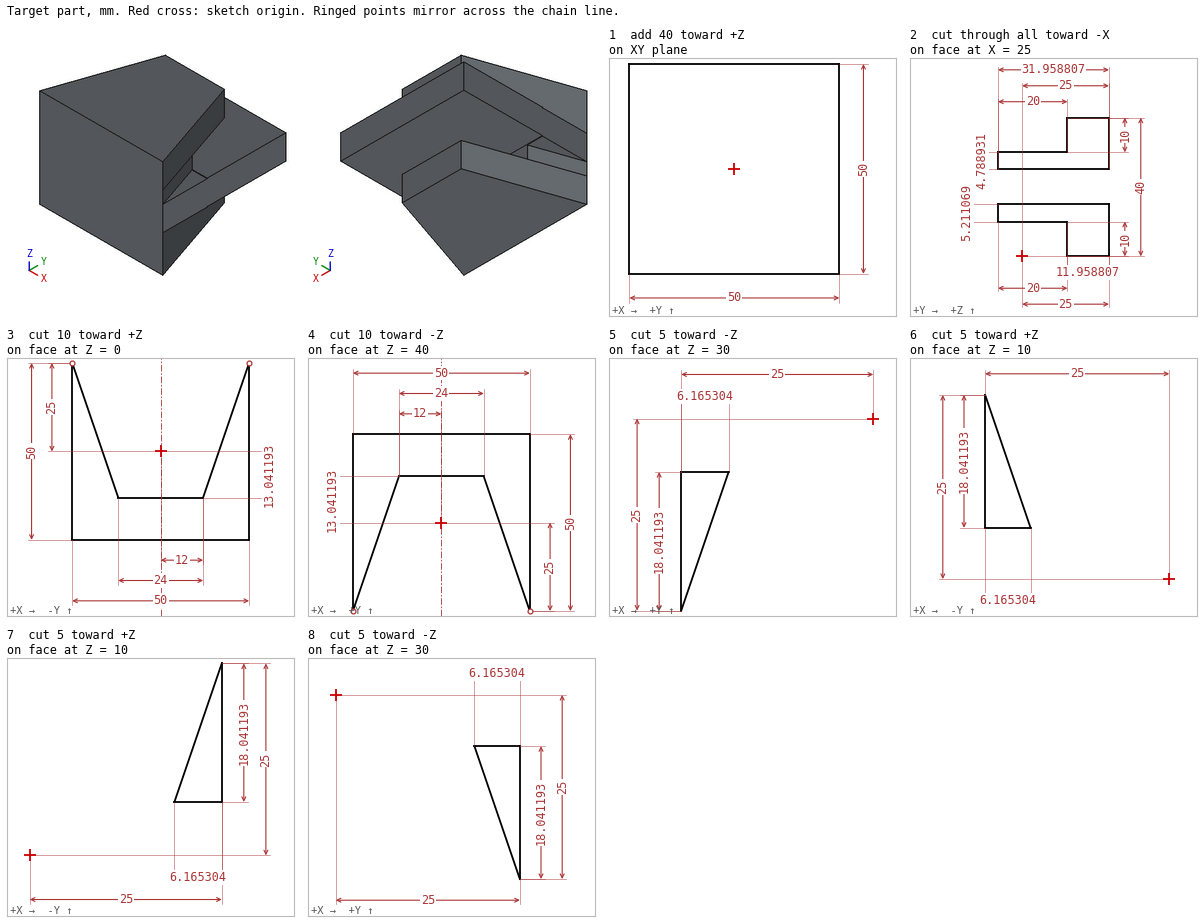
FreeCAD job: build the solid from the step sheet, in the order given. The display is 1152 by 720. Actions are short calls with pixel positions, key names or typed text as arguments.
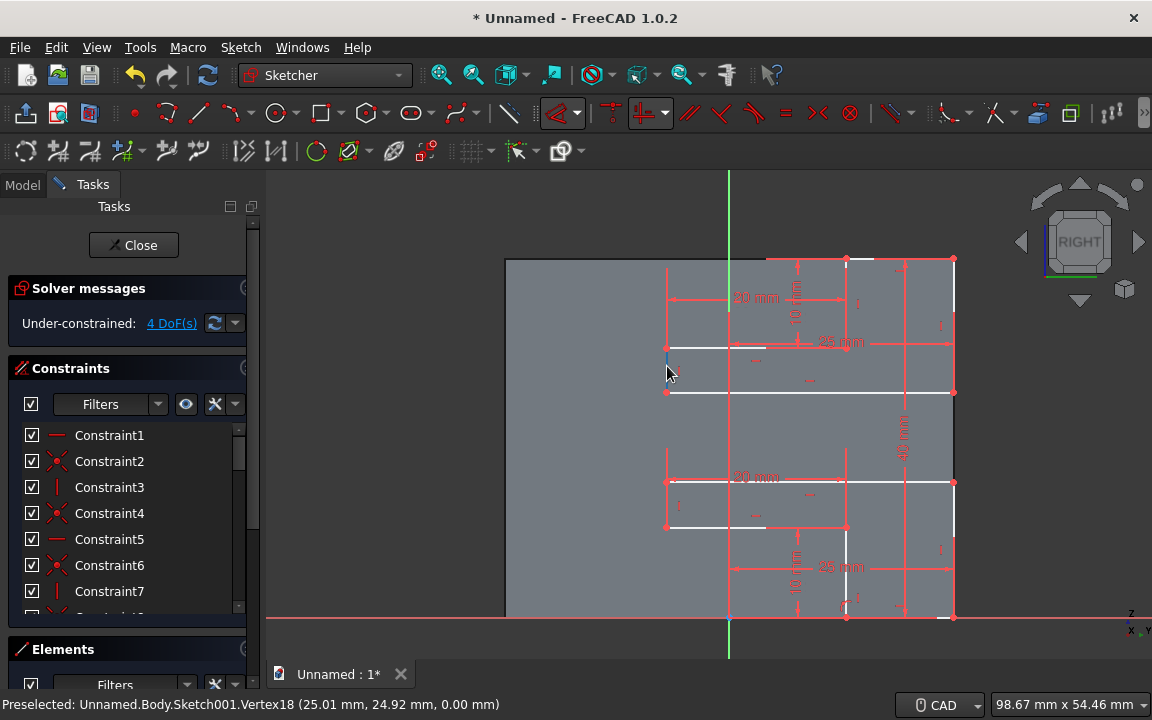
click(667, 366)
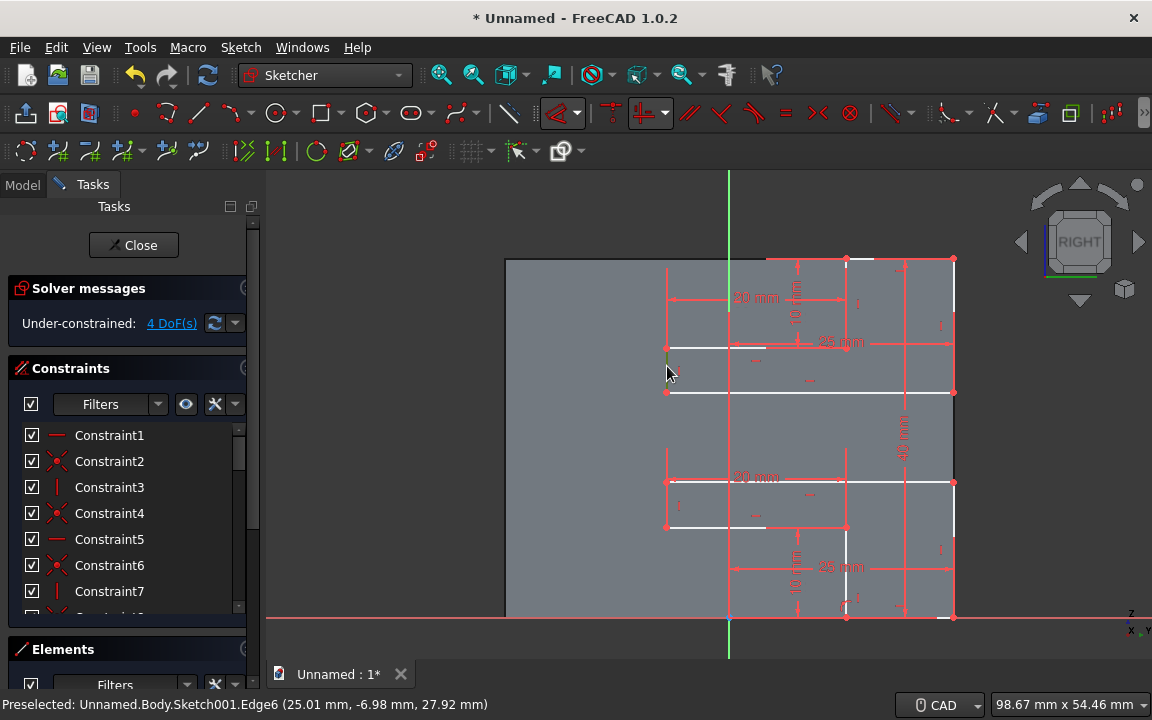
key(i)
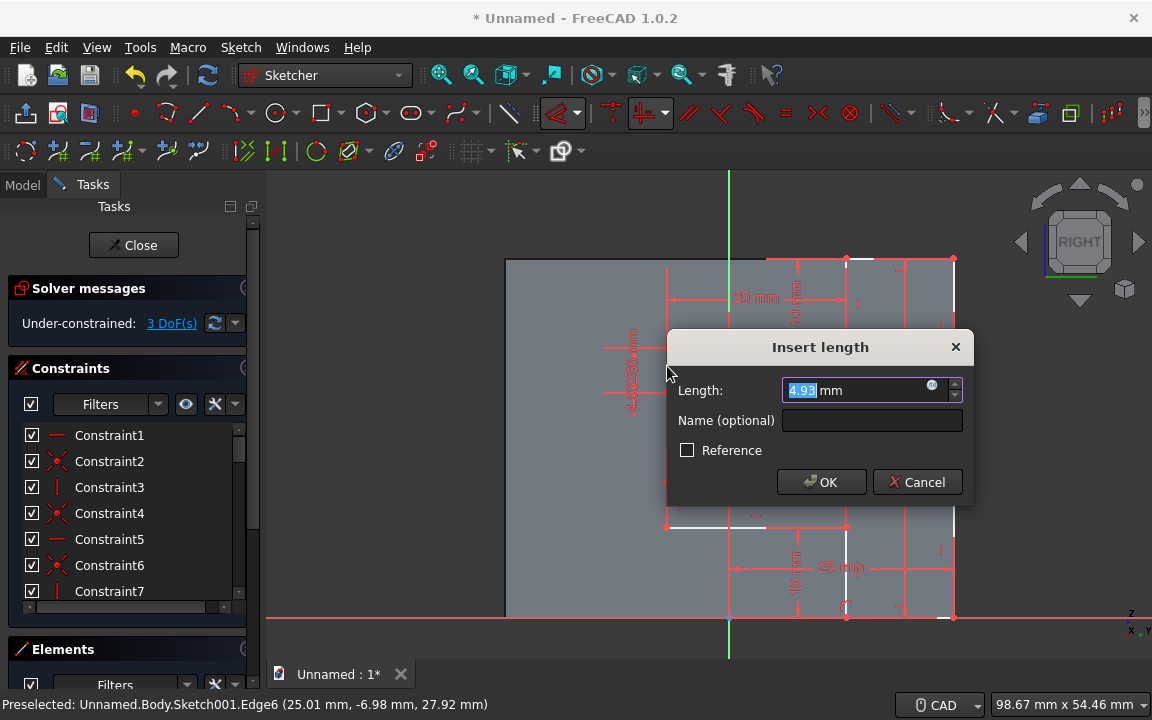
text(4.788931)
key(Return)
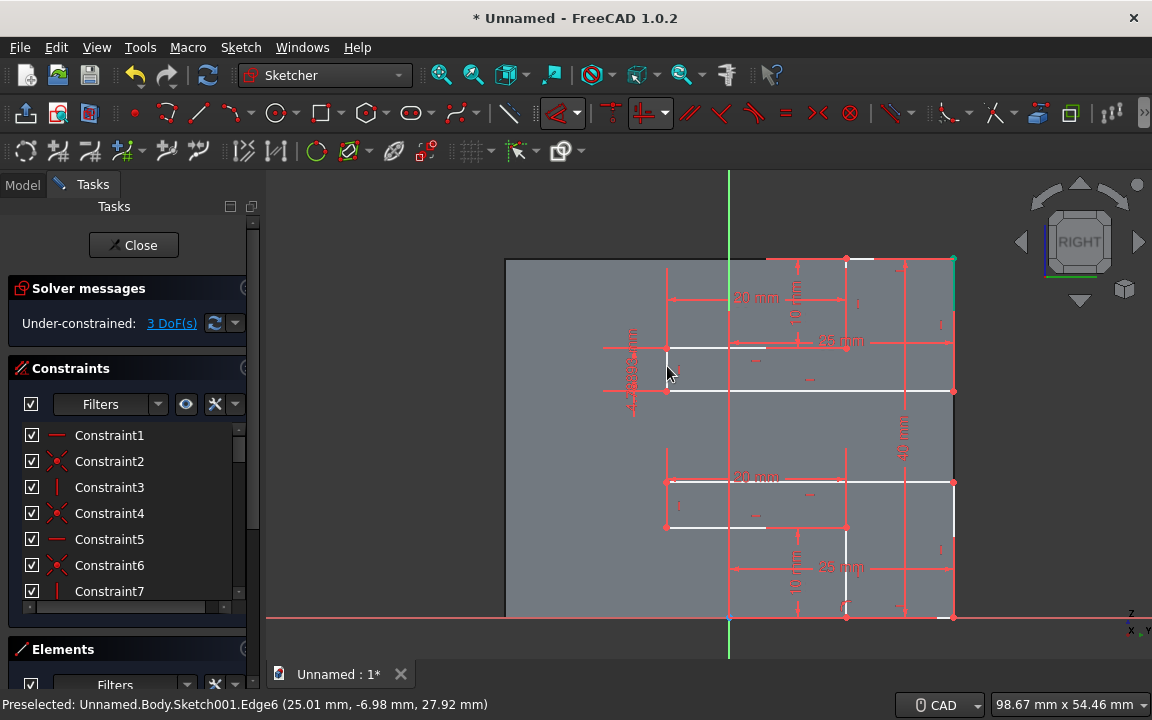
click(667, 496)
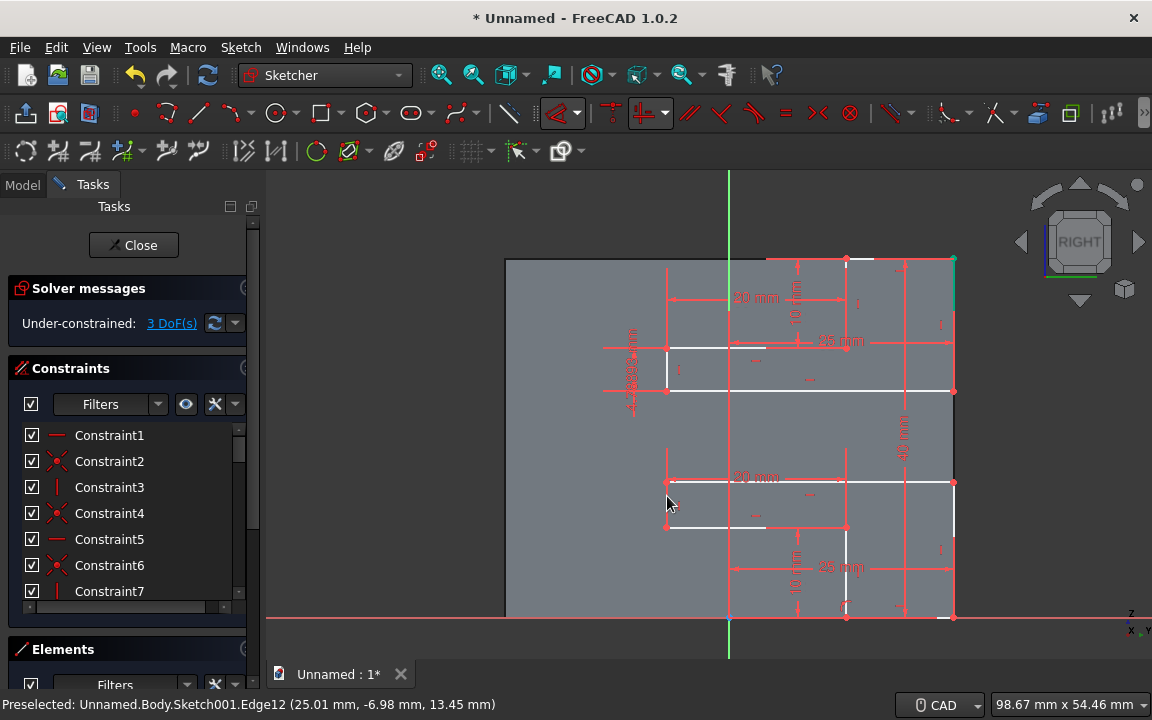
key(i)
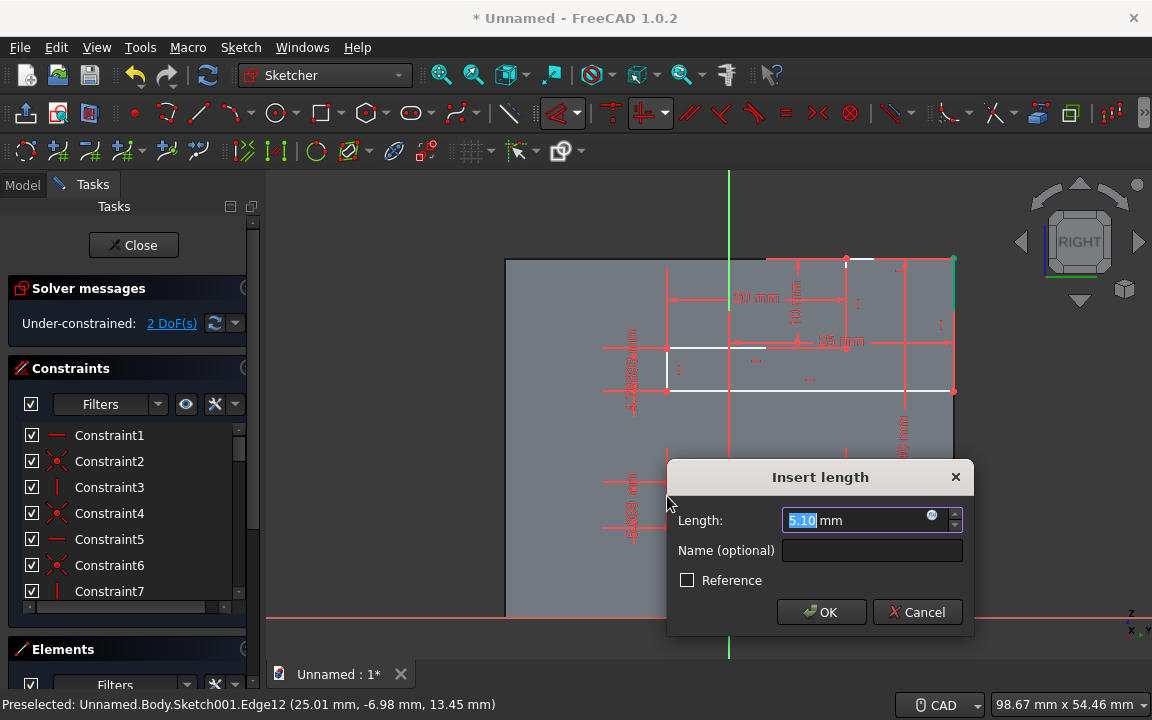
text(5.211069)
key(Return)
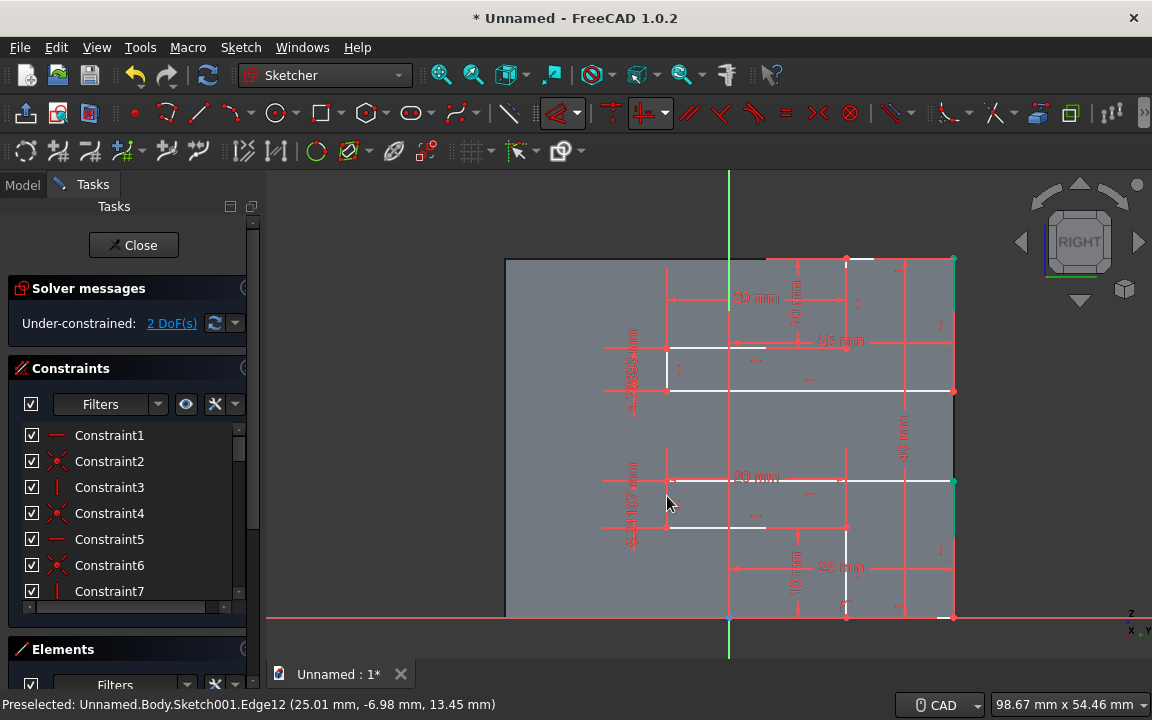
click(753, 391)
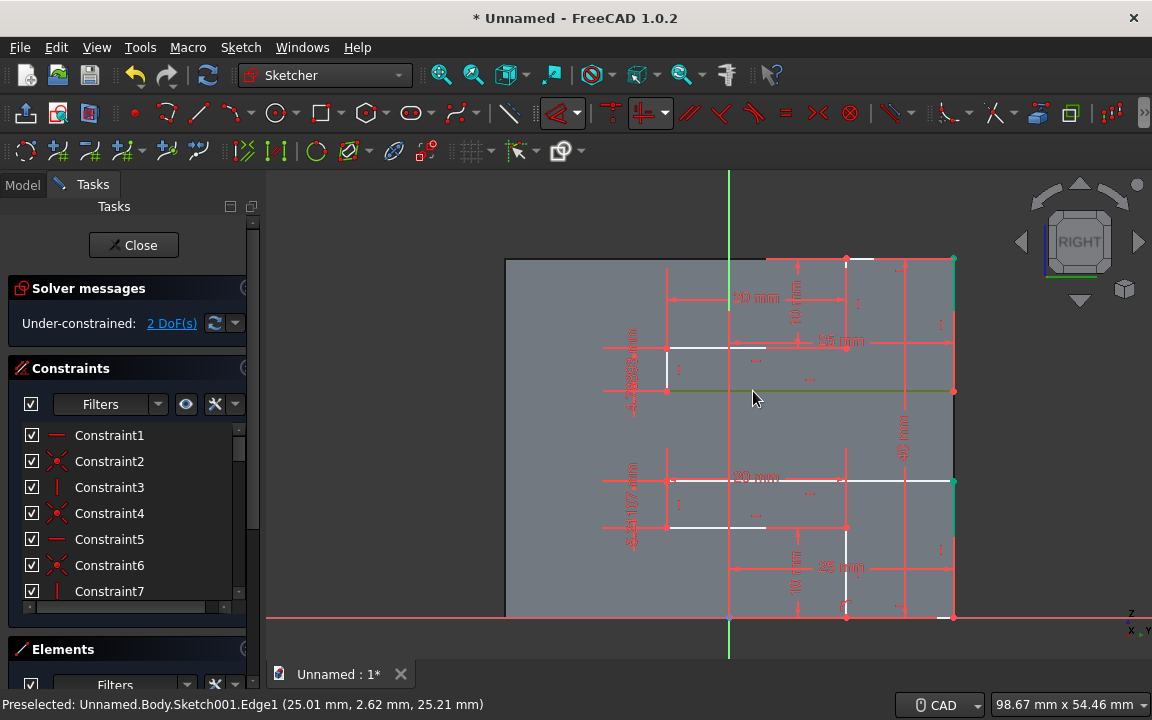
key(l)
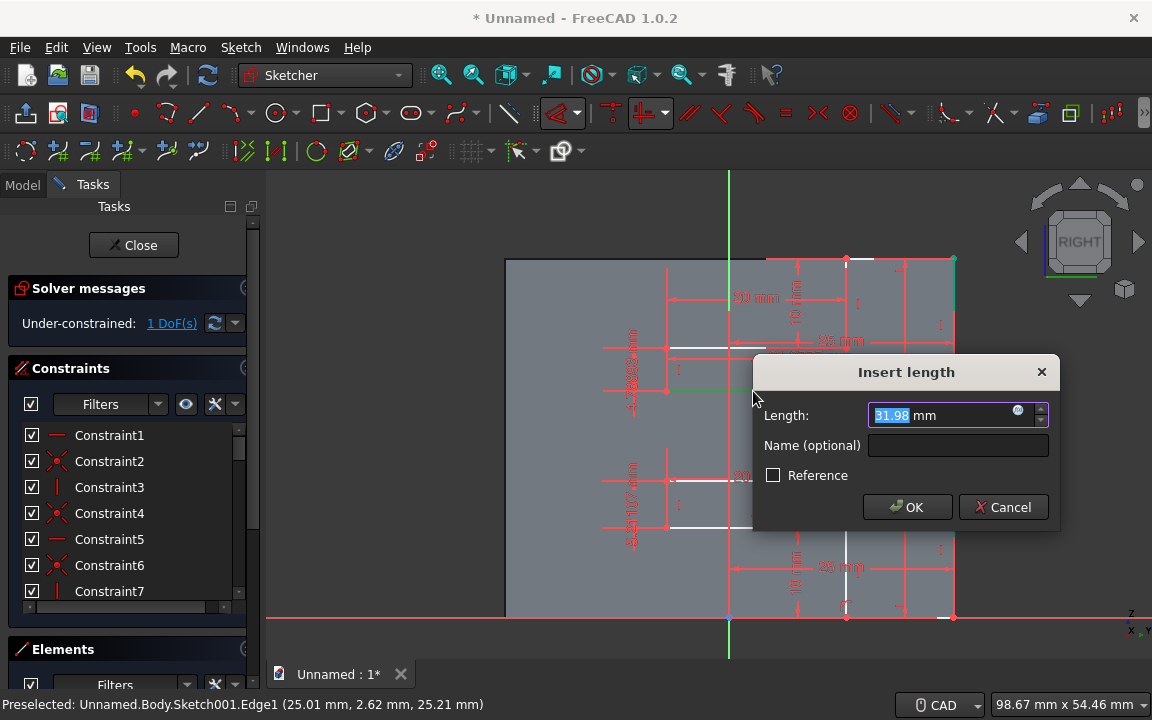
text(31.958807)
key(Return)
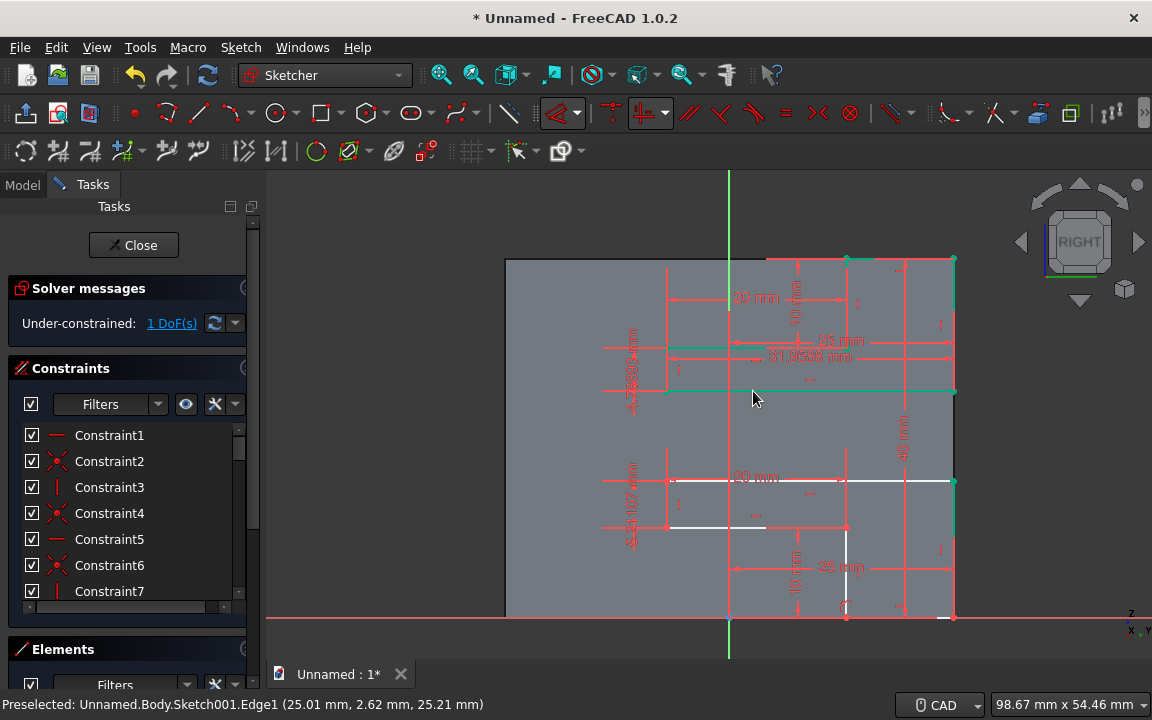
click(879, 618)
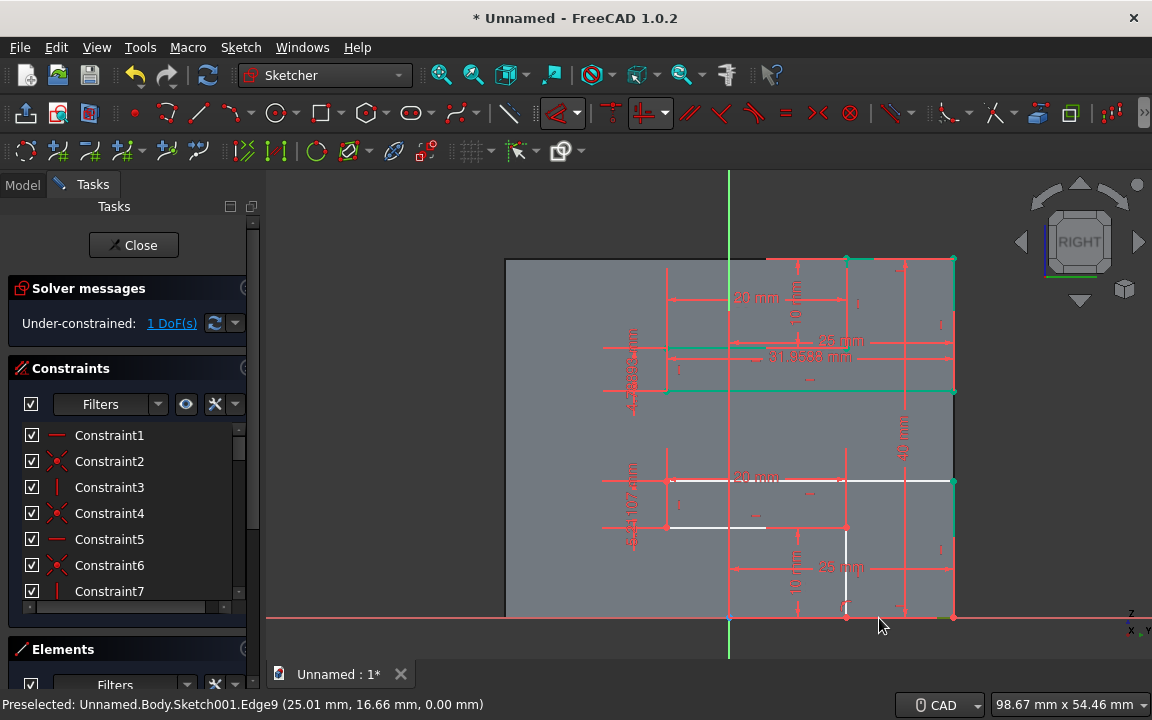
key(l)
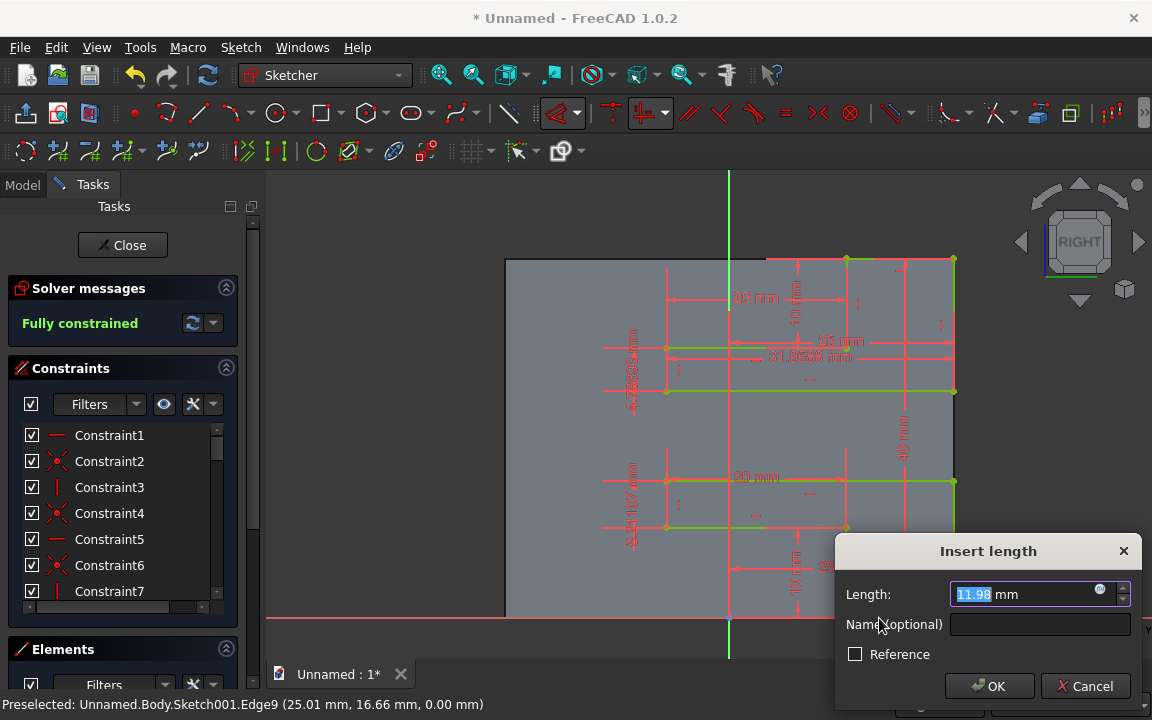
text(11.958807)
key(Return)